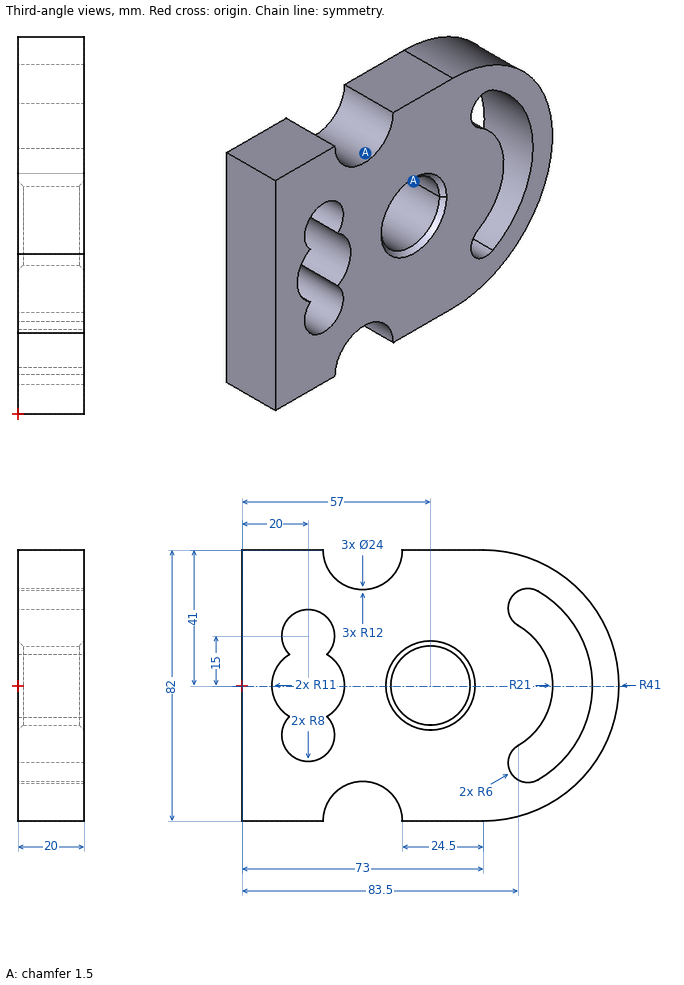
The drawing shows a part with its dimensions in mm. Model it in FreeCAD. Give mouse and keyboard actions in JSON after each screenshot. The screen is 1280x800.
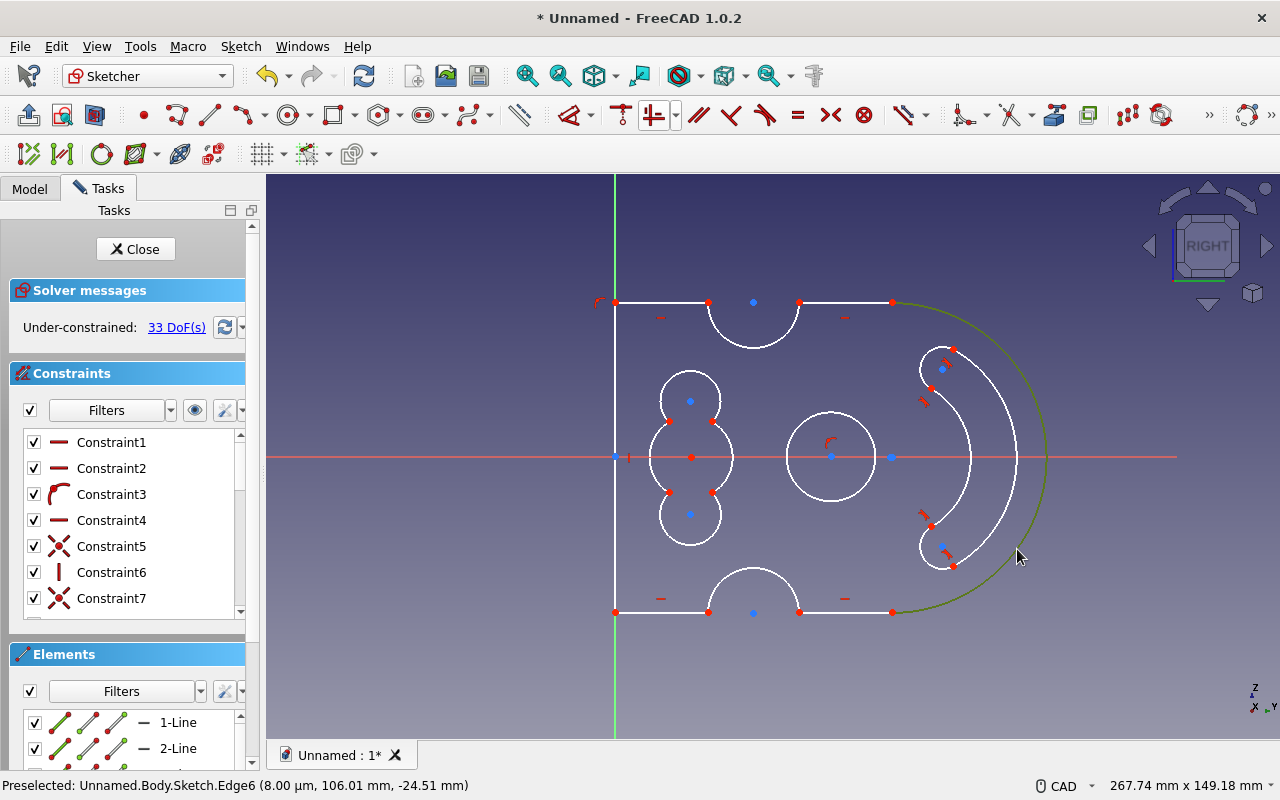
{"action": "left_click", "coordinate": [964, 490]}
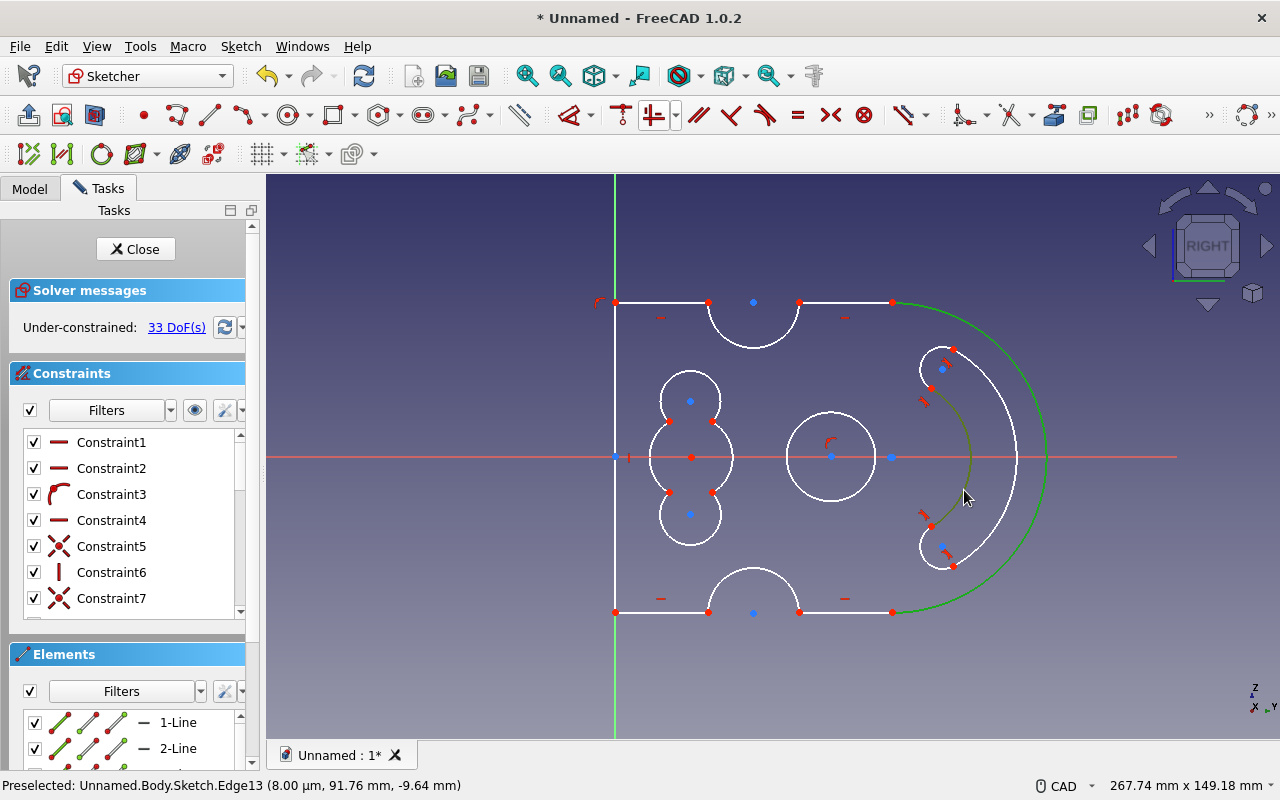
{"action": "left_click", "coordinate": [621, 116]}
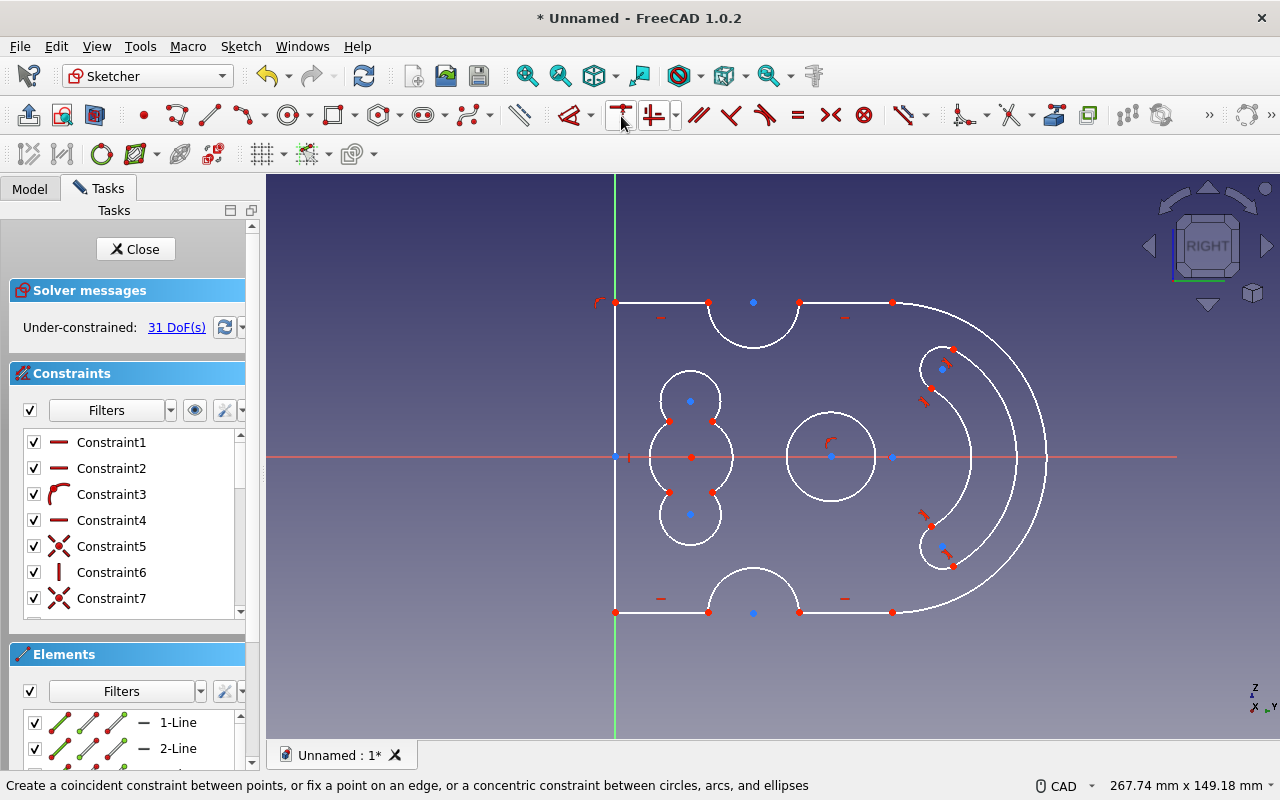
{"action": "left_click", "coordinate": [1017, 549]}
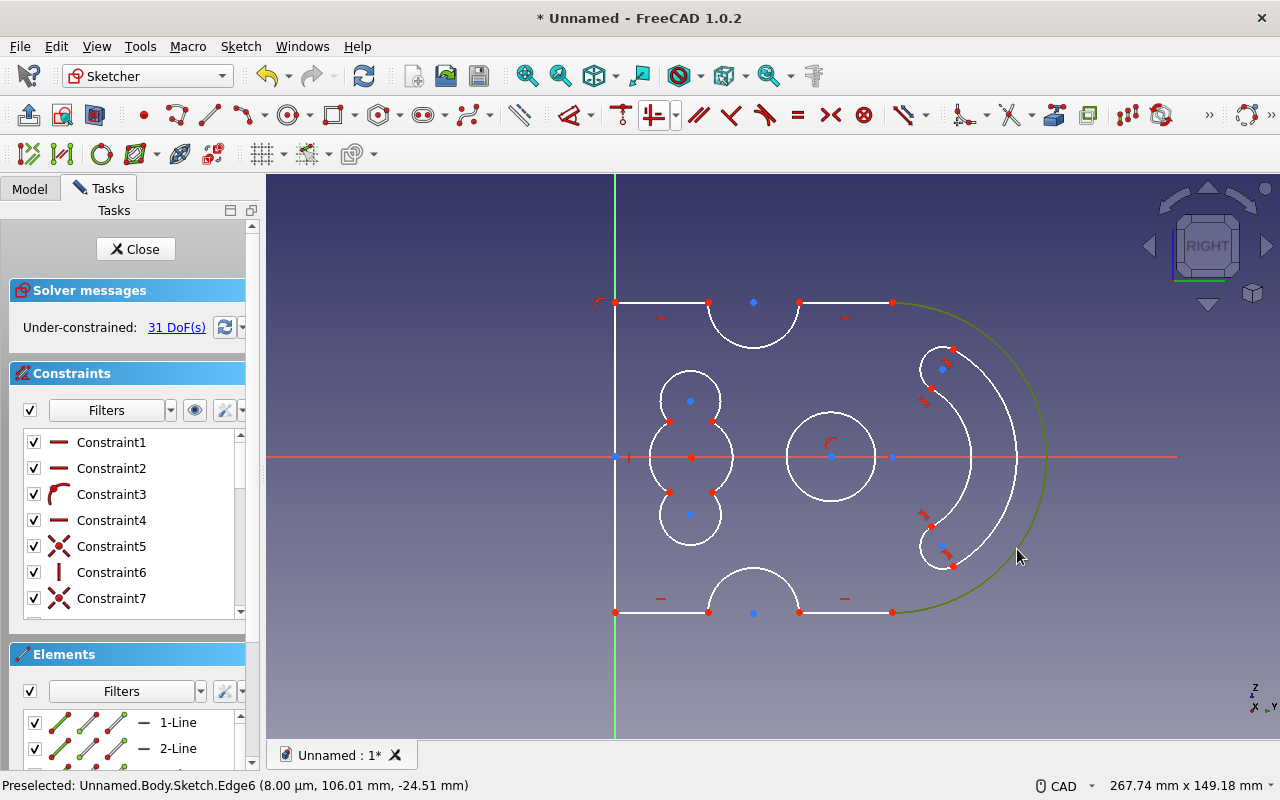
{"action": "left_click", "coordinate": [1006, 509]}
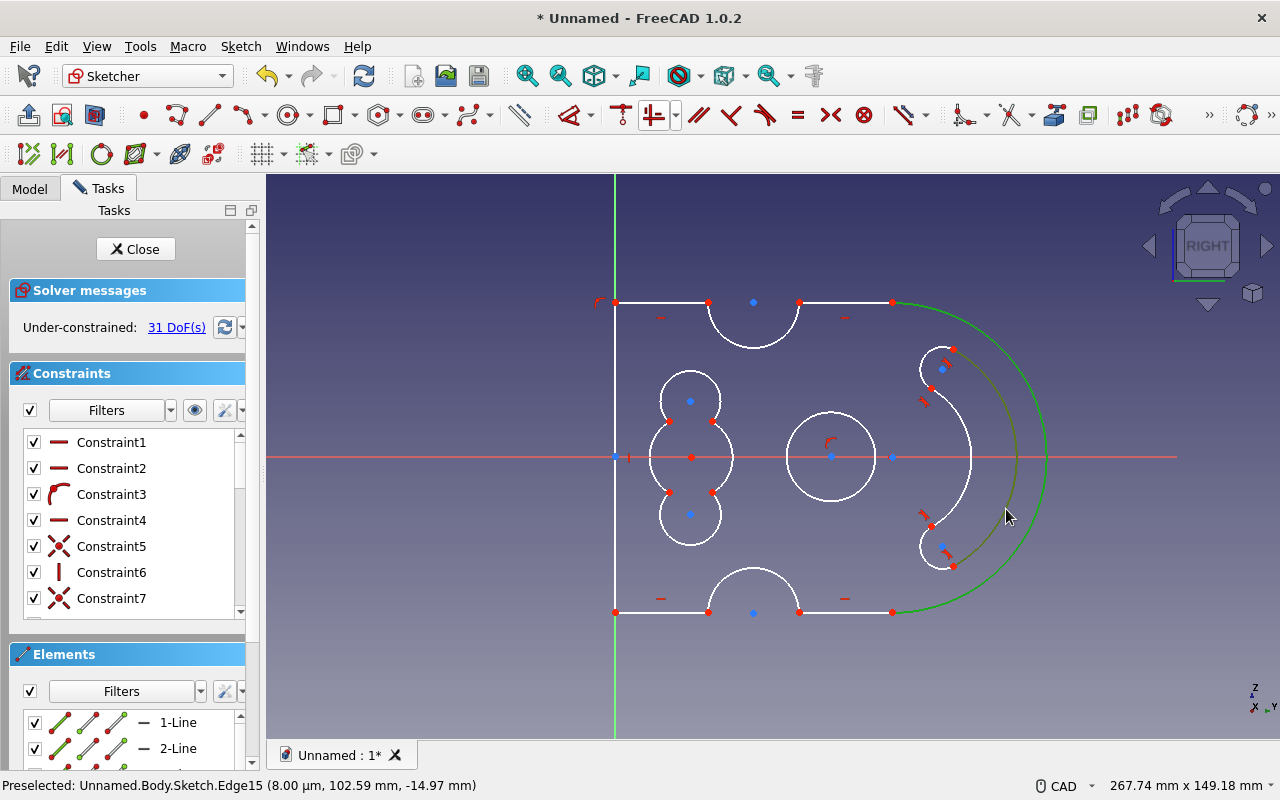
{"action": "key", "text": "c"}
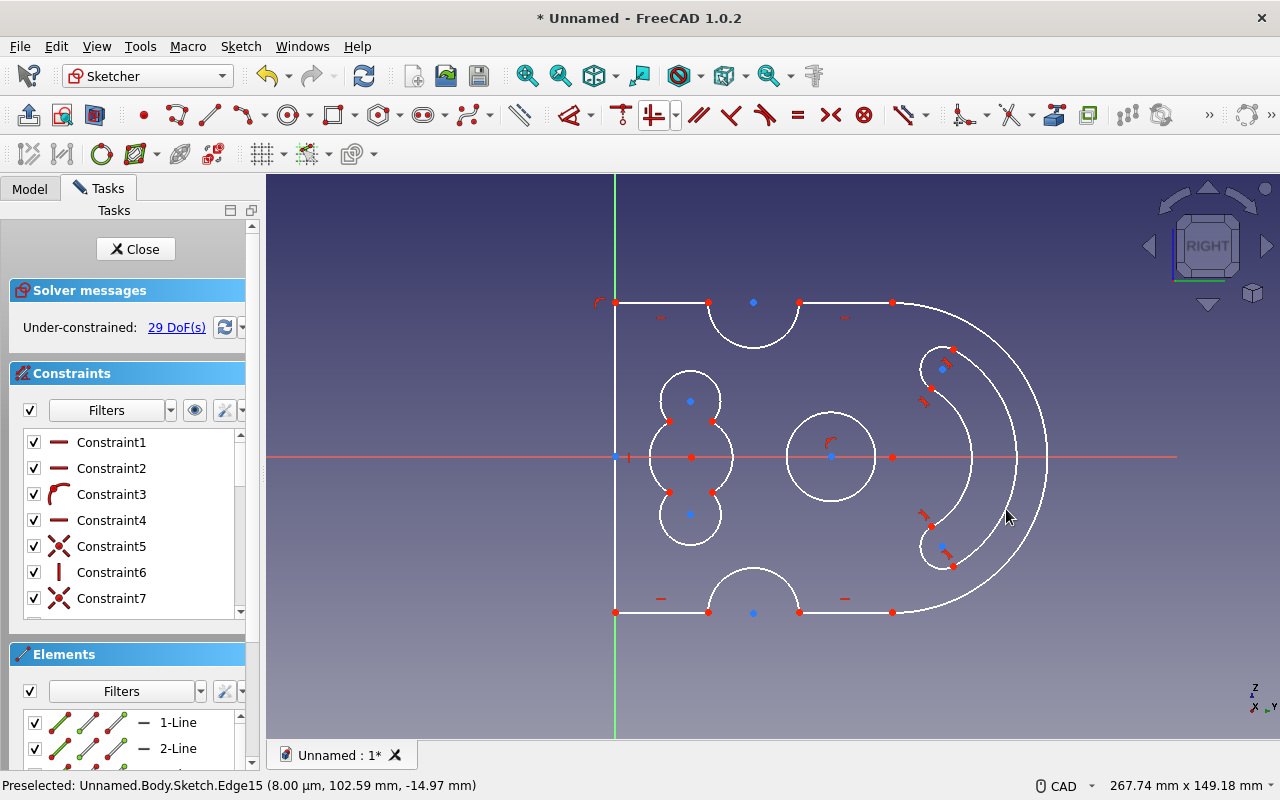
{"action": "left_click", "coordinate": [727, 339]}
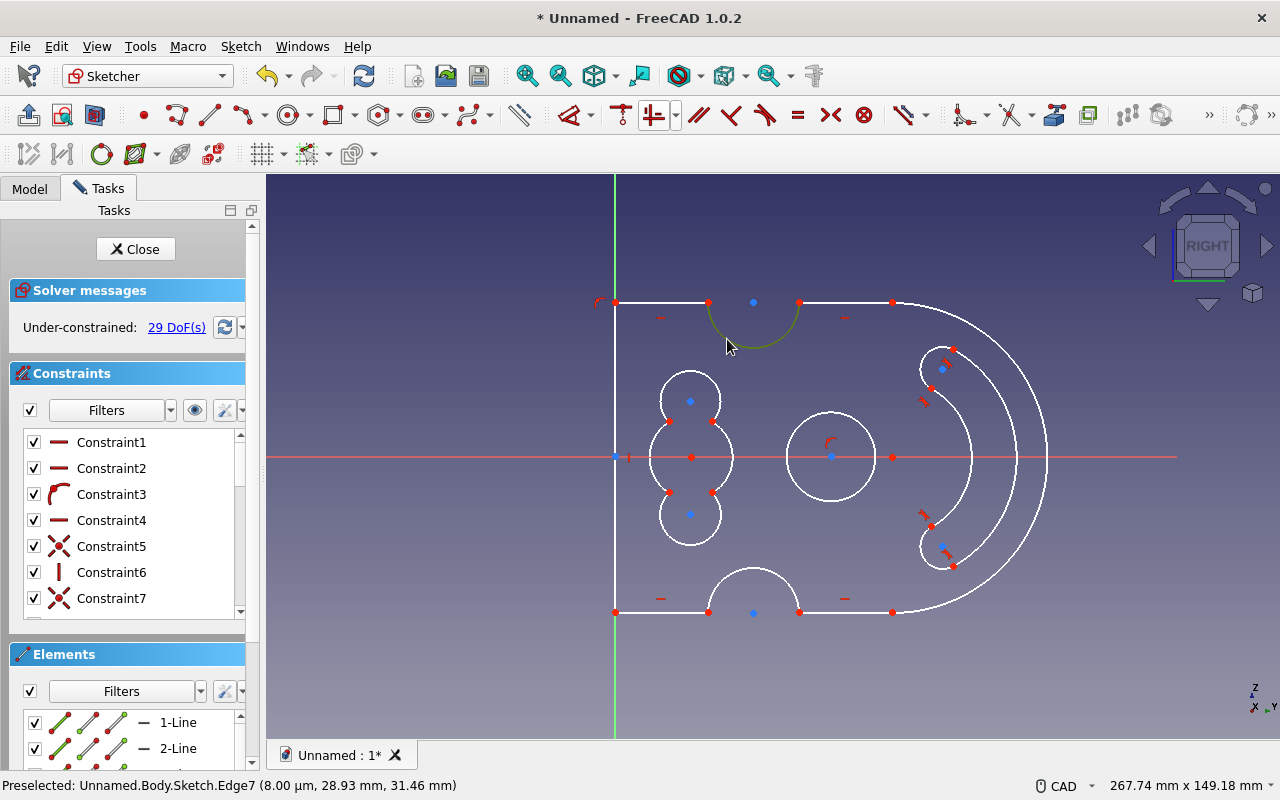
{"action": "left_click", "coordinate": [780, 577]}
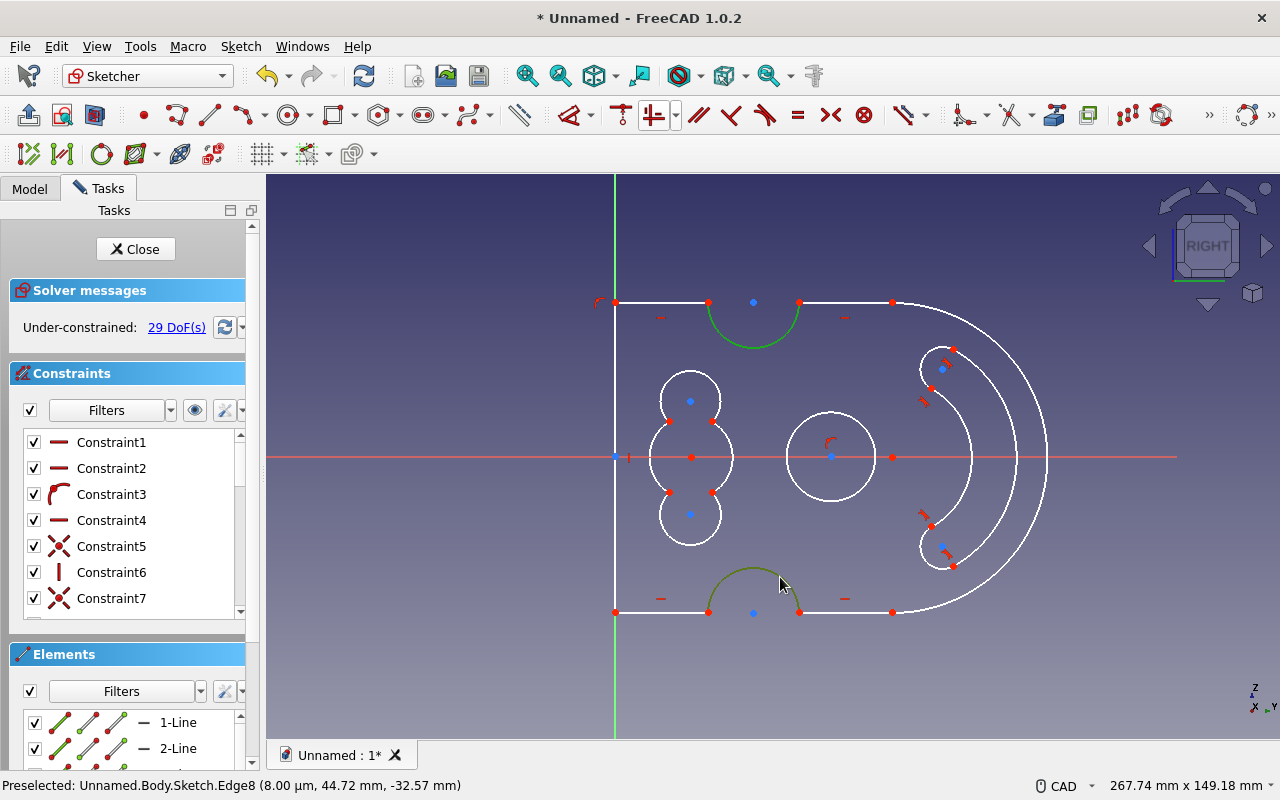
{"action": "key", "text": "e"}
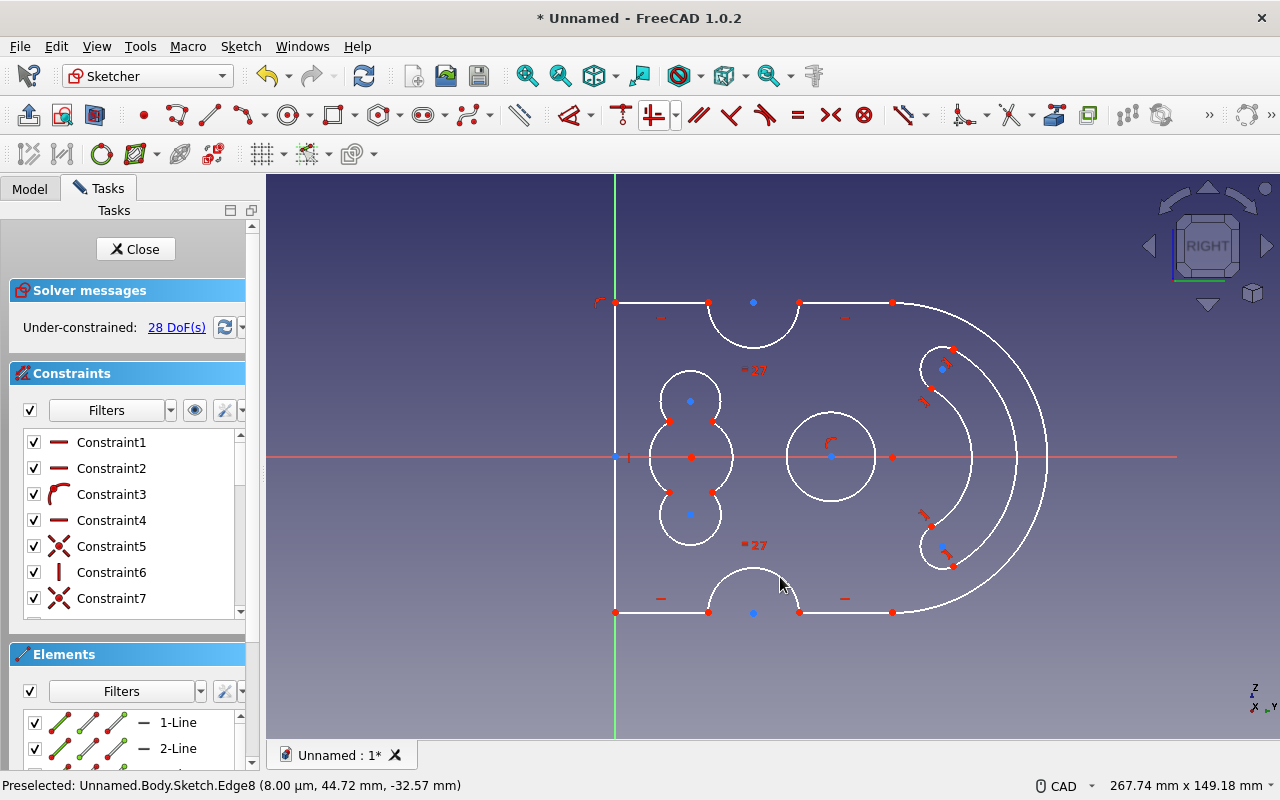
{"action": "left_click", "coordinate": [653, 441]}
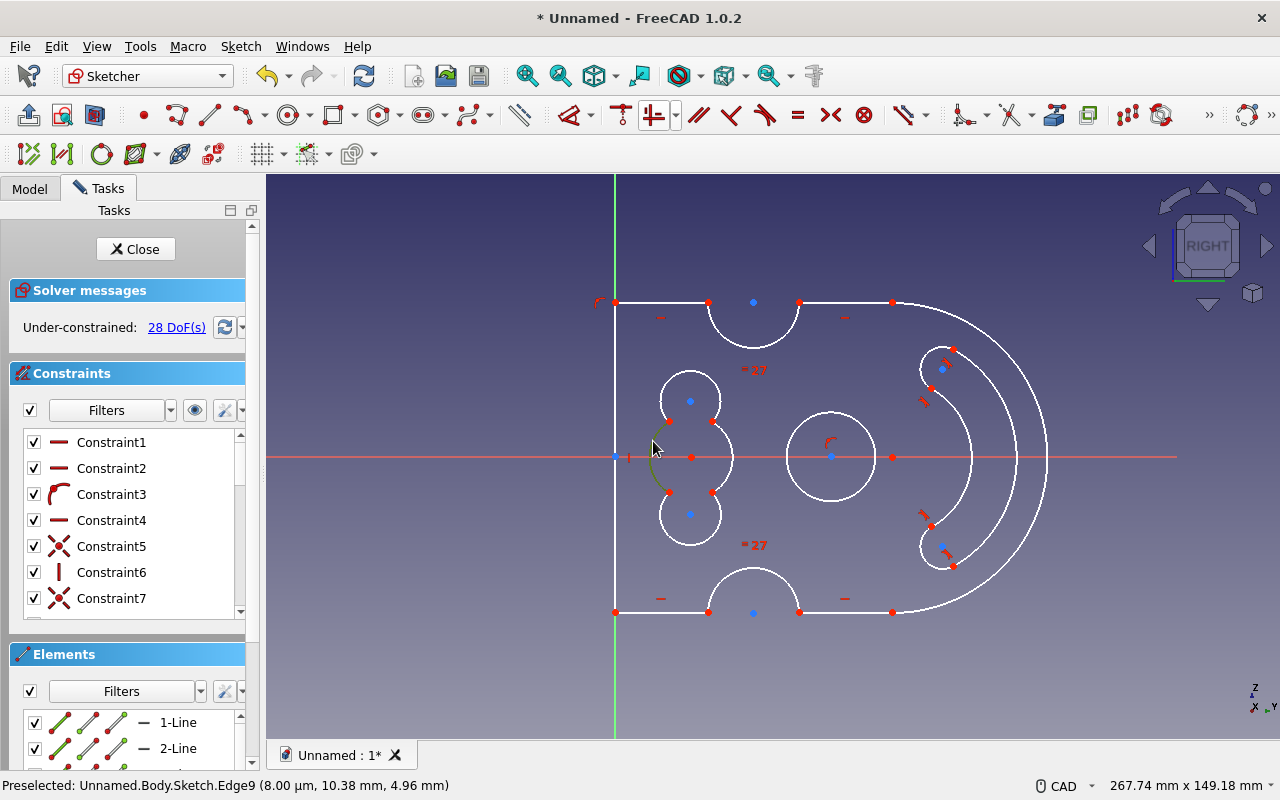
{"action": "left_click", "coordinate": [729, 474]}